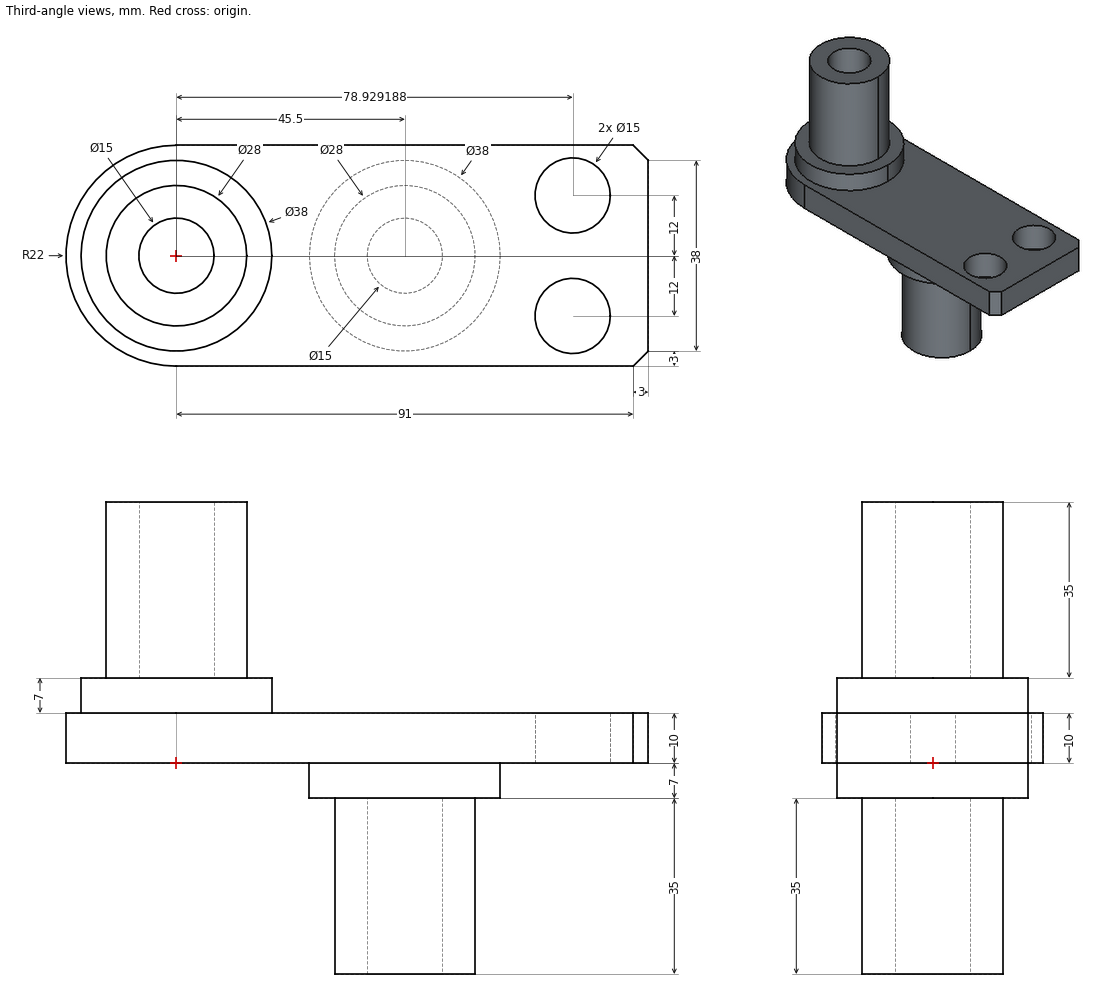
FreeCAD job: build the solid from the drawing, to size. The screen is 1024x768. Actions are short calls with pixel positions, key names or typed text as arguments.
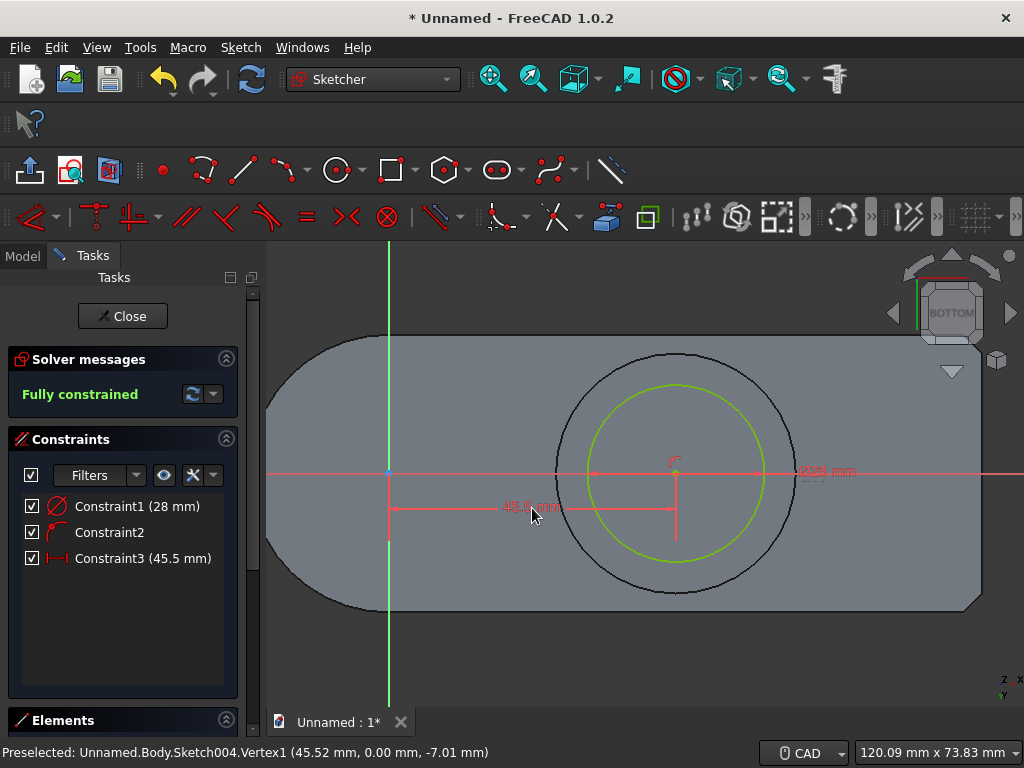
click(123, 316)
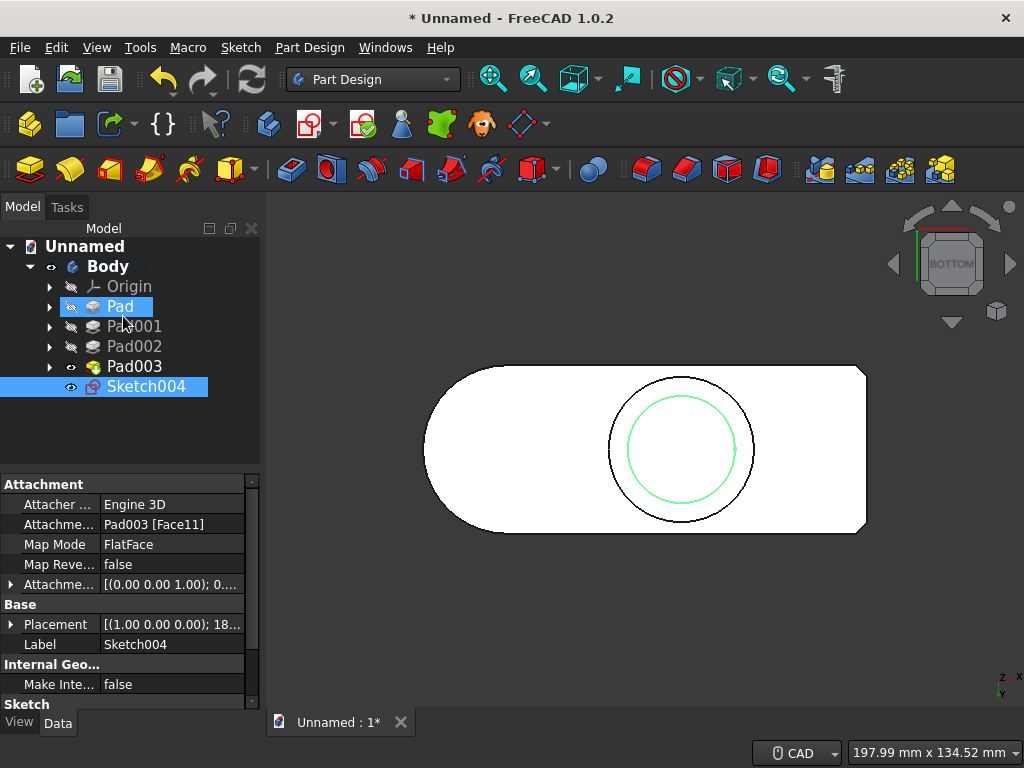
click(30, 170)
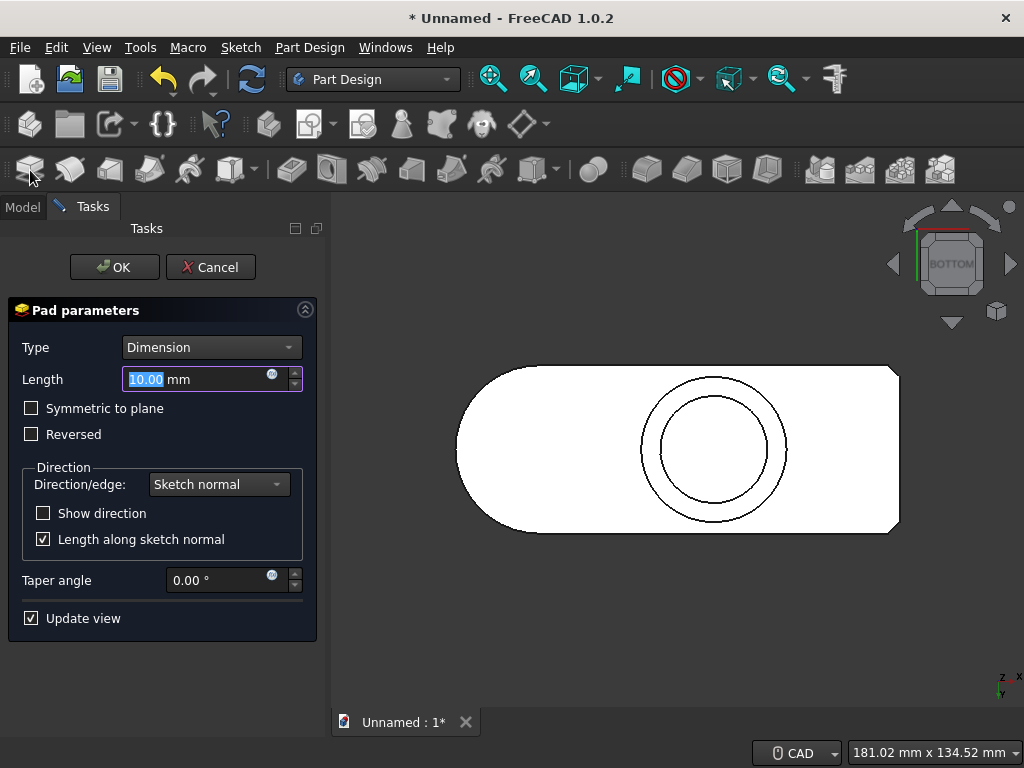
text(35)
key(Tab)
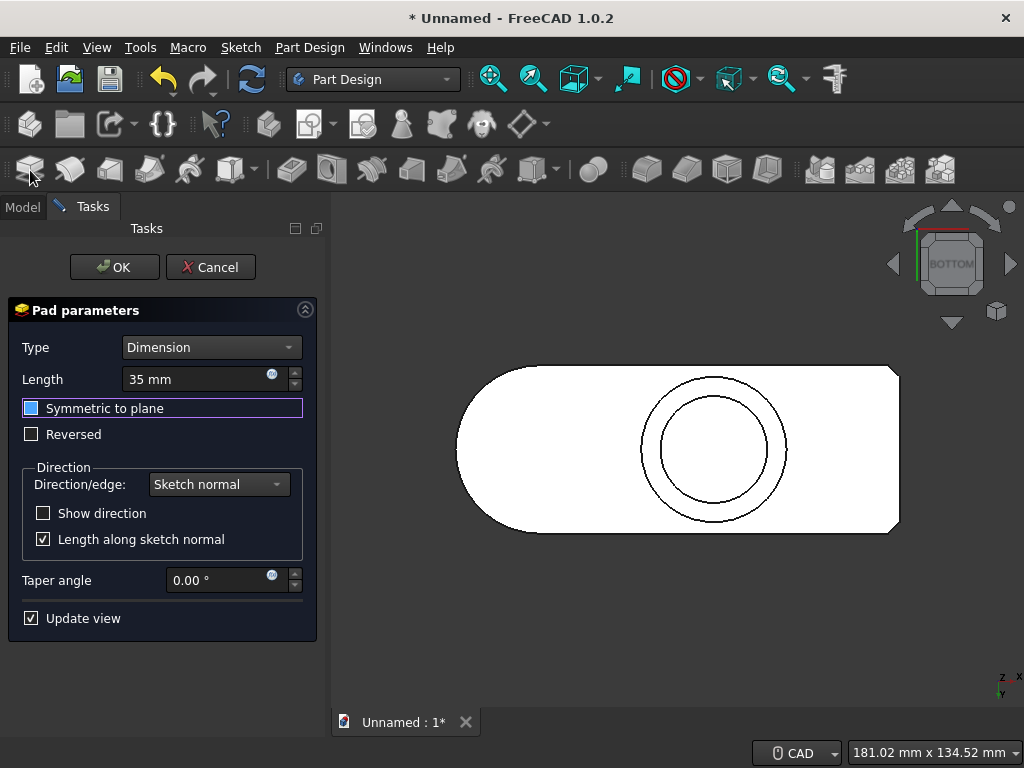
click(115, 267)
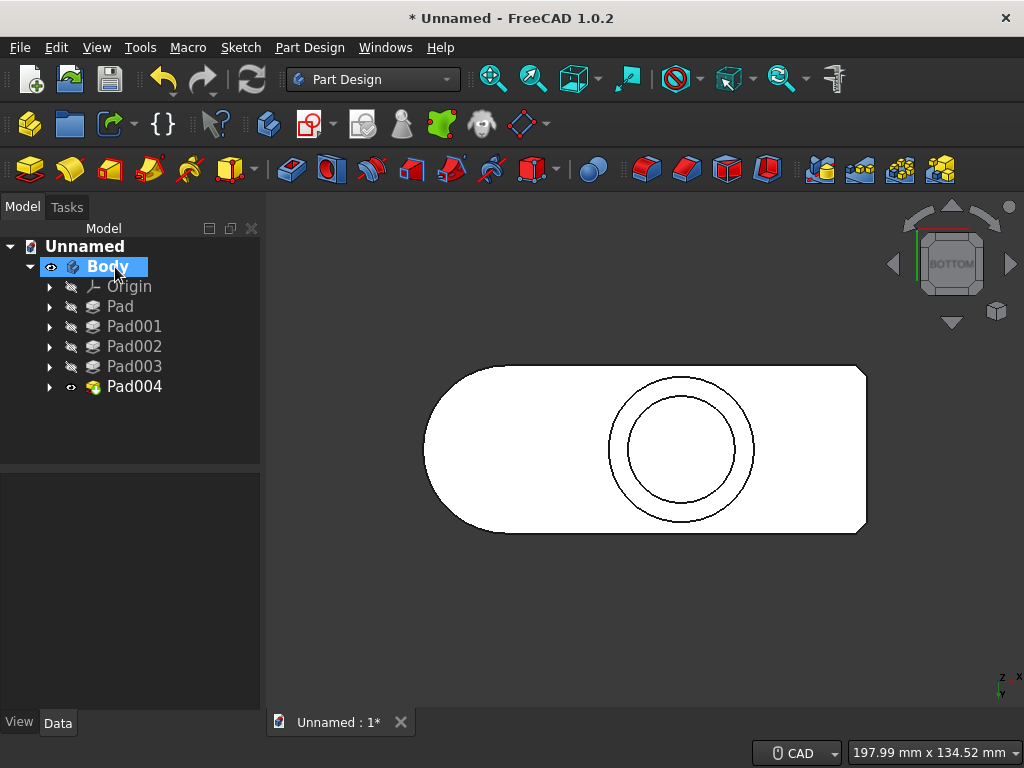
click(681, 448)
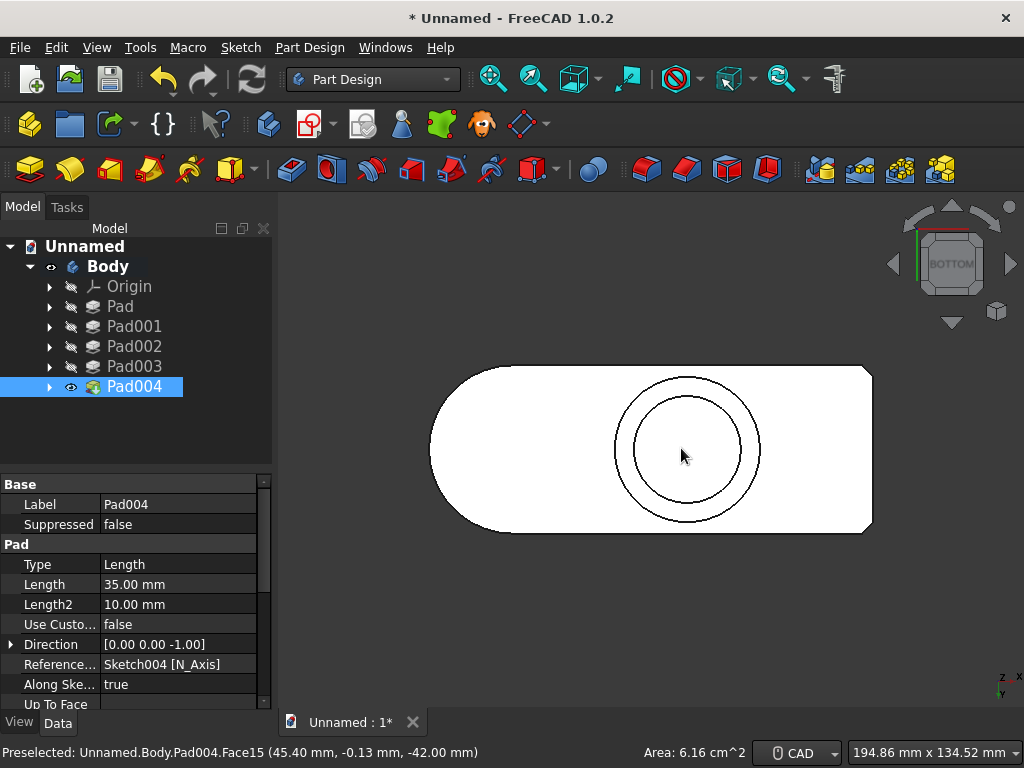
click(310, 124)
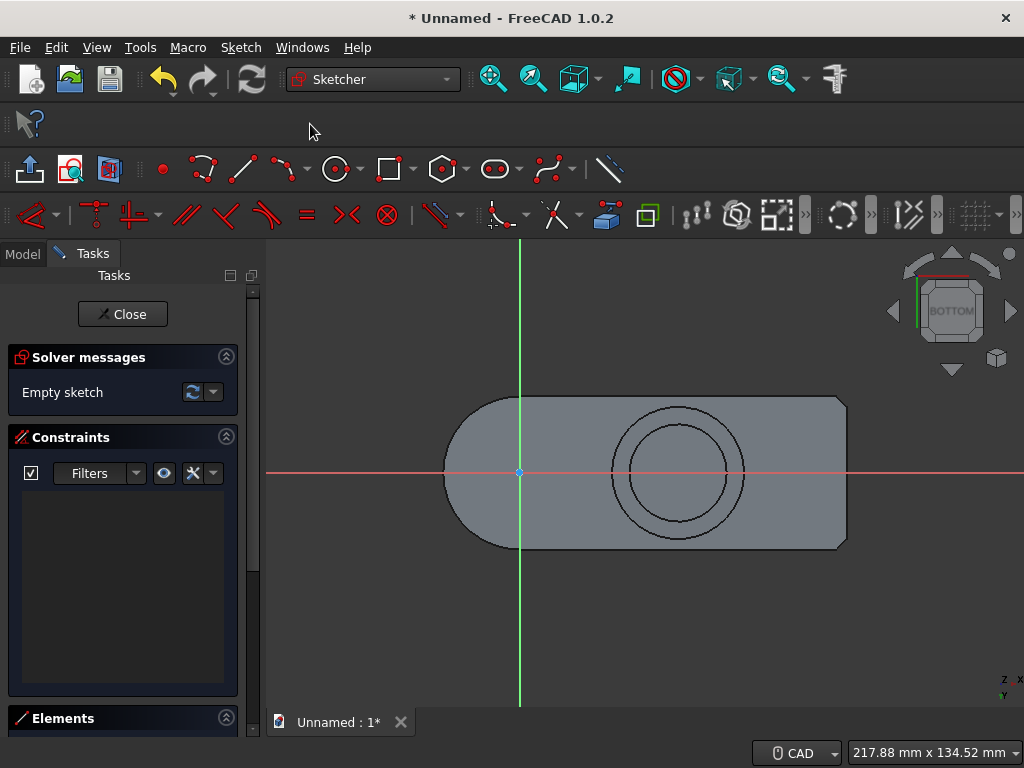
scroll(698, 473, up, 9)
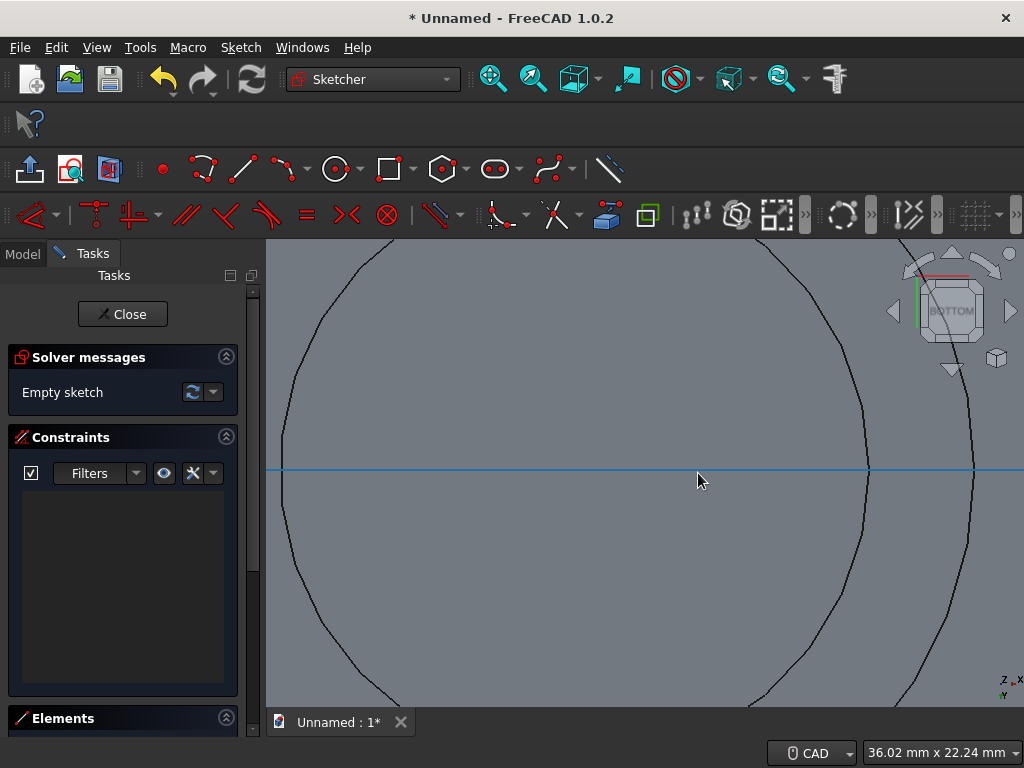
click(336, 170)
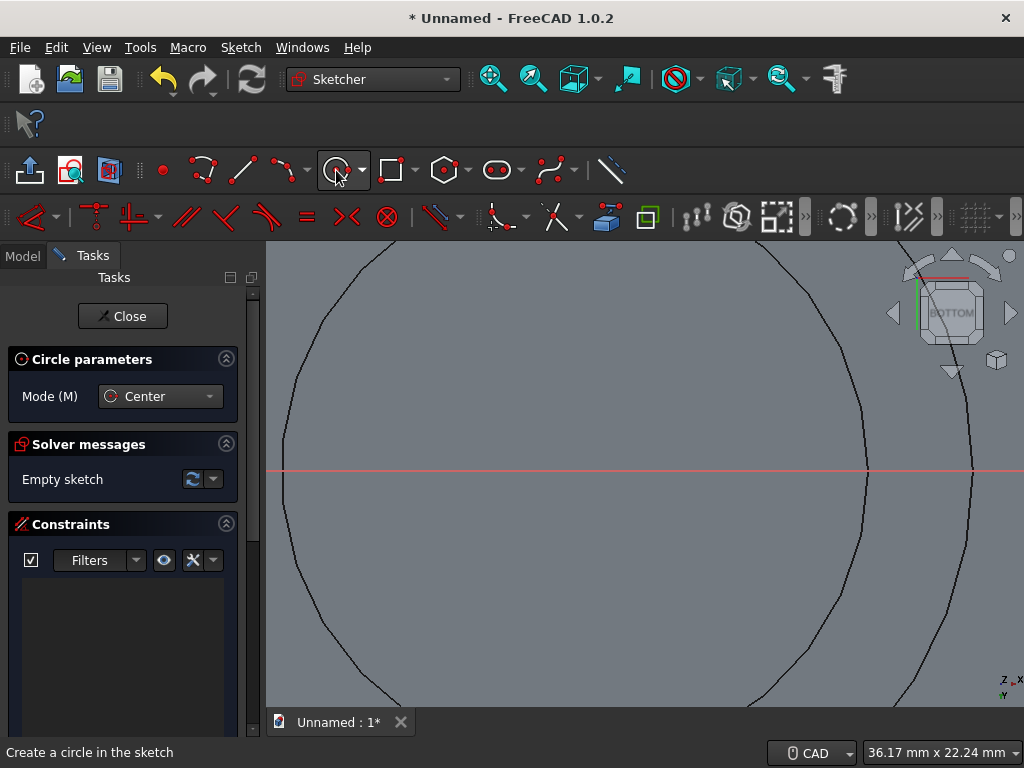
click(575, 471)
move(686, 360)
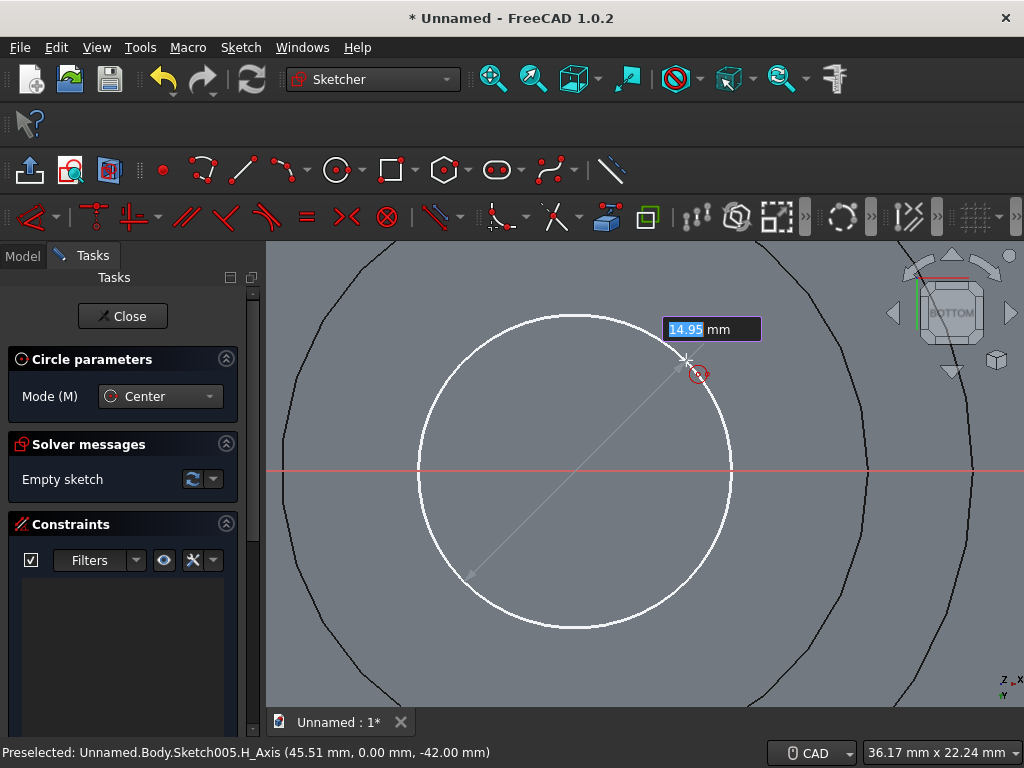
text(15)
key(Return)
key(Escape)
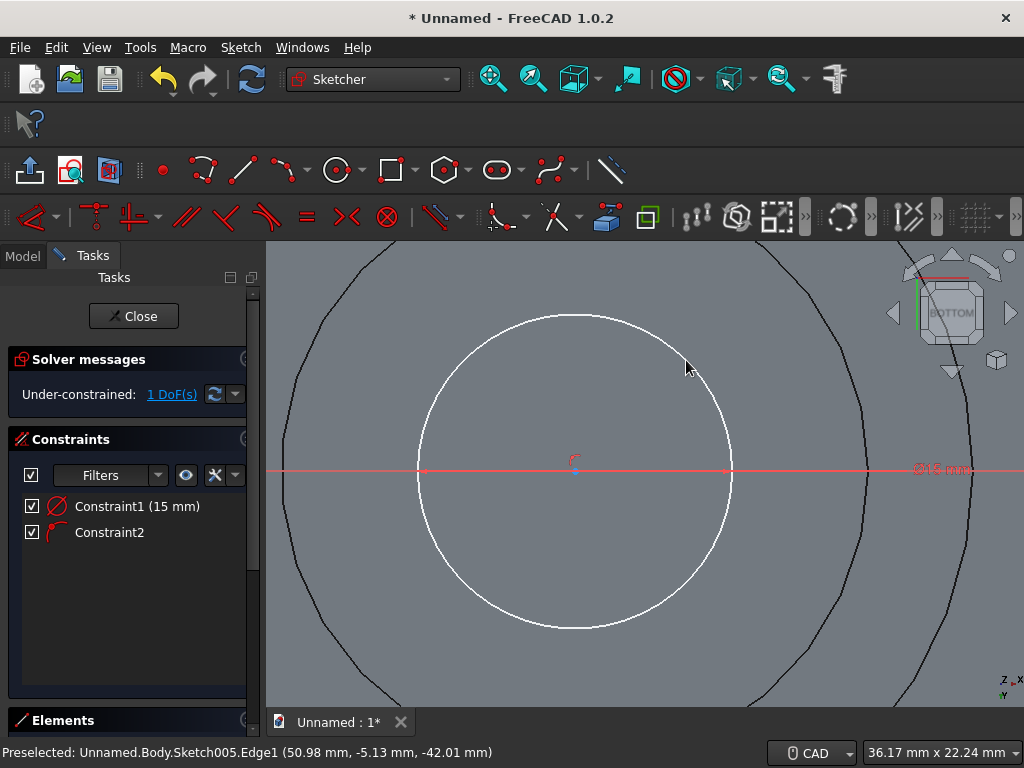
click(32, 218)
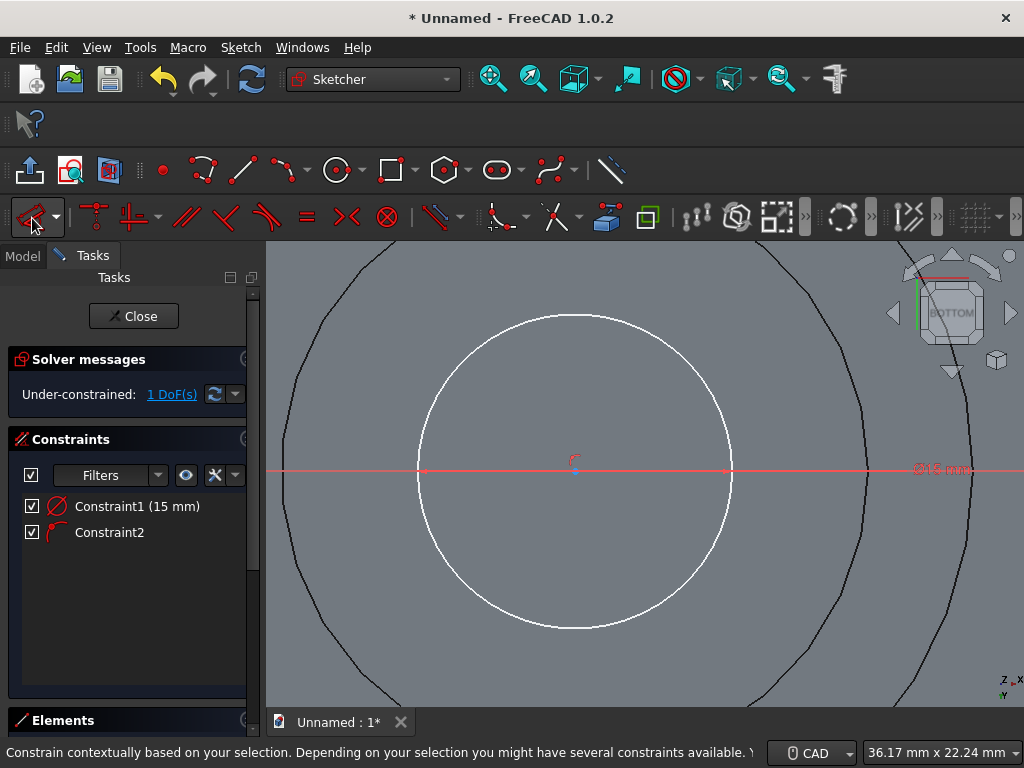
click(575, 471)
click(370, 505)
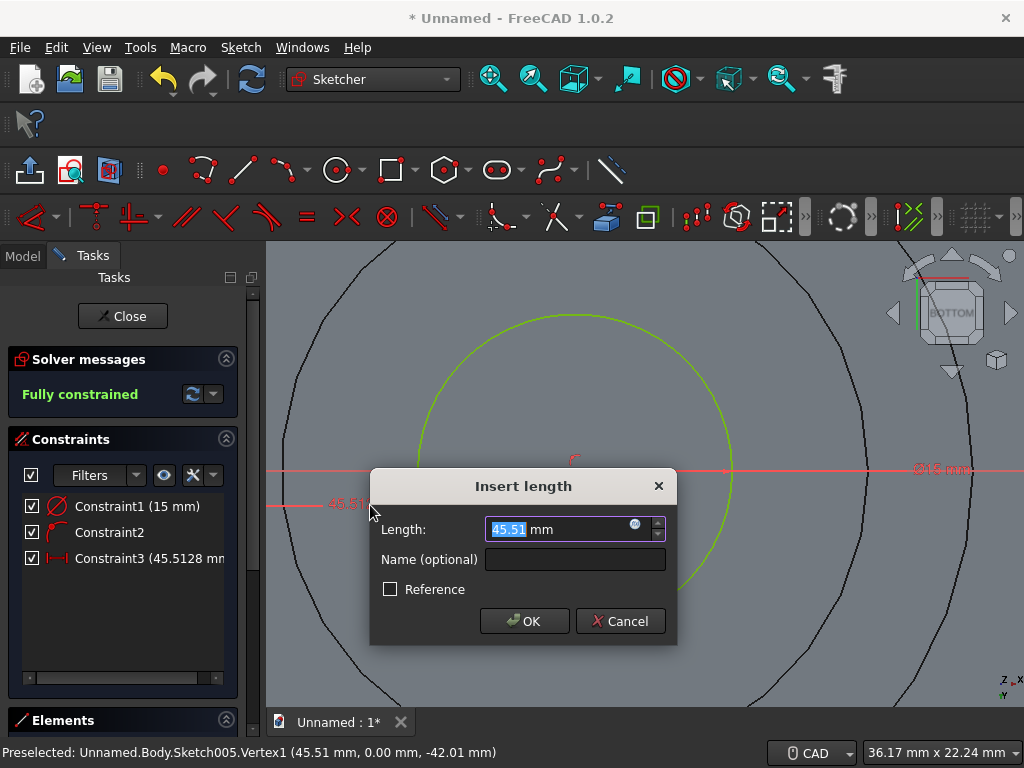
text(45.5)
key(Return)
key(Escape)